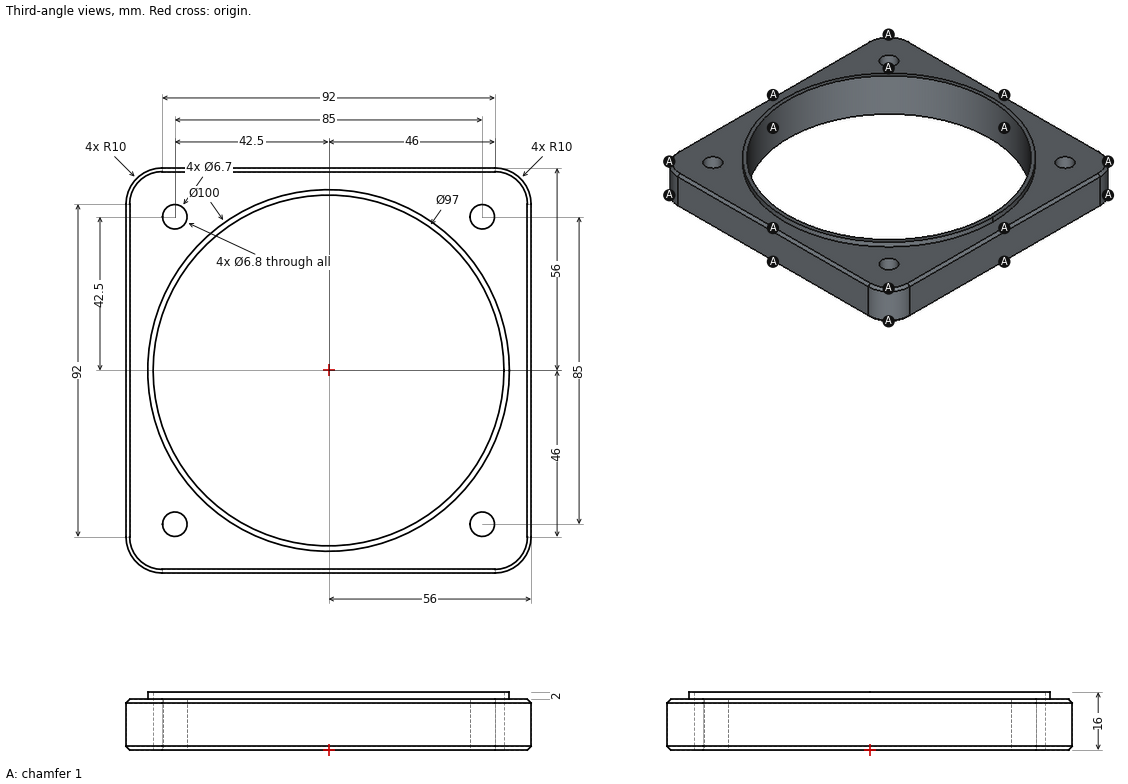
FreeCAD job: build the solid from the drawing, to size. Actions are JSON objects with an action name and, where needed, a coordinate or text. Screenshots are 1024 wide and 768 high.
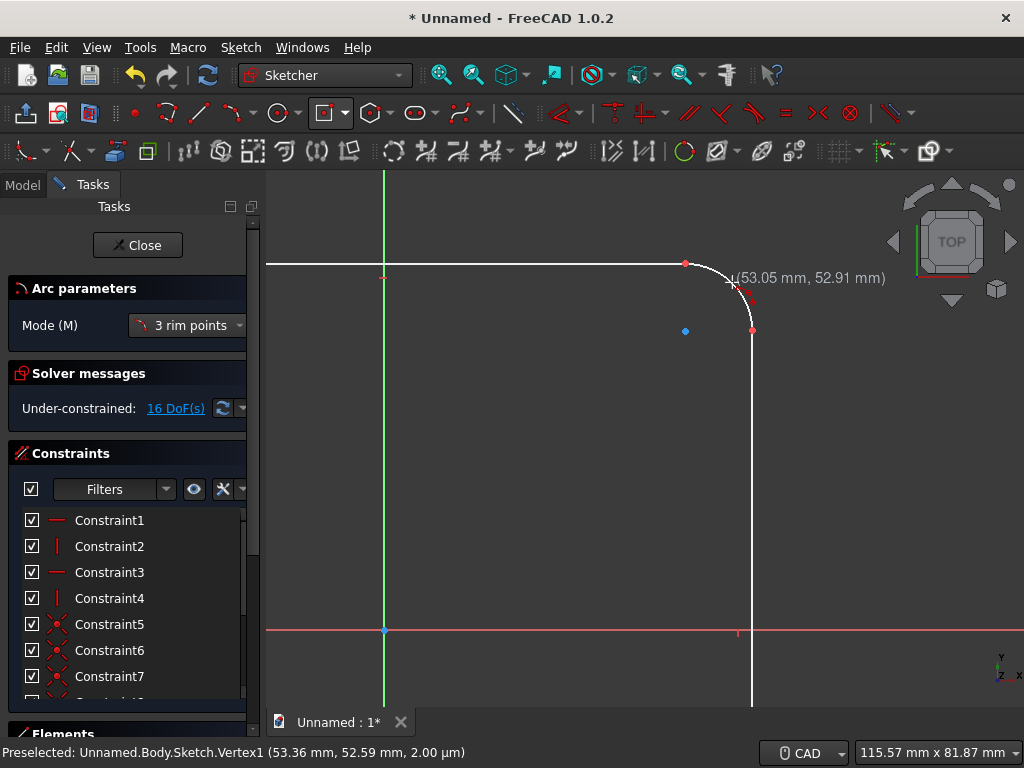
{"action": "left_click", "coordinate": [278, 114]}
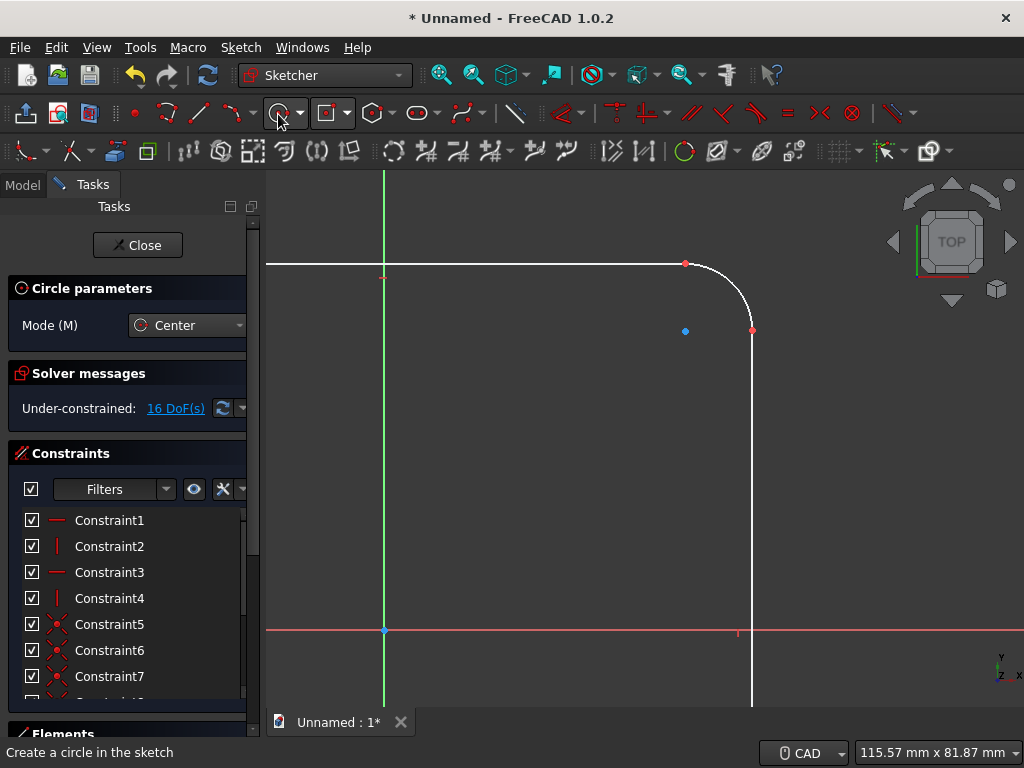
{"action": "left_click", "coordinate": [384, 630]}
{"action": "mouse_move", "coordinate": [609, 405]}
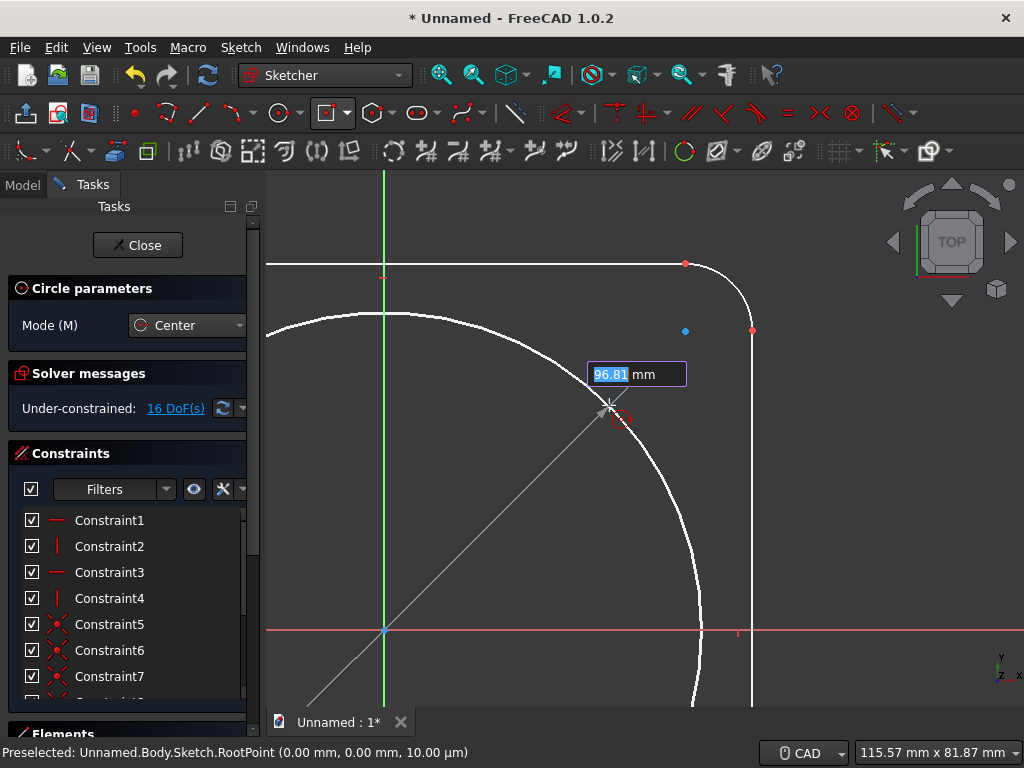
{"action": "type", "text": "97"}
{"action": "key", "text": "Return"}
{"action": "key", "text": "Escape"}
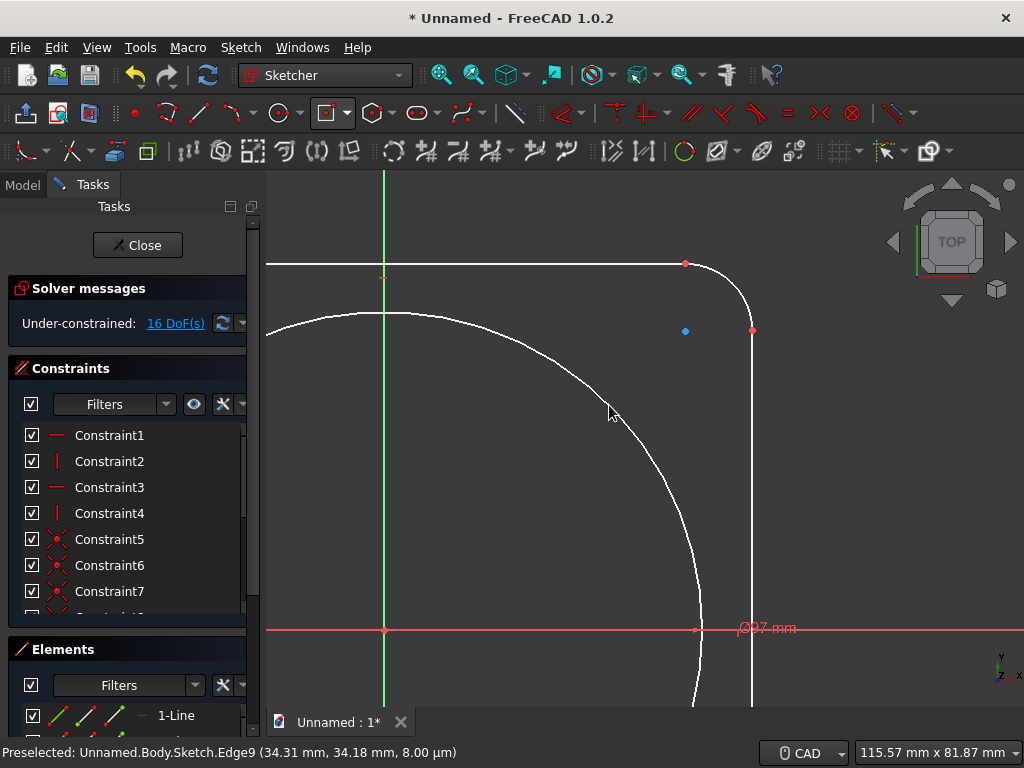
{"action": "left_click", "coordinate": [505, 264]}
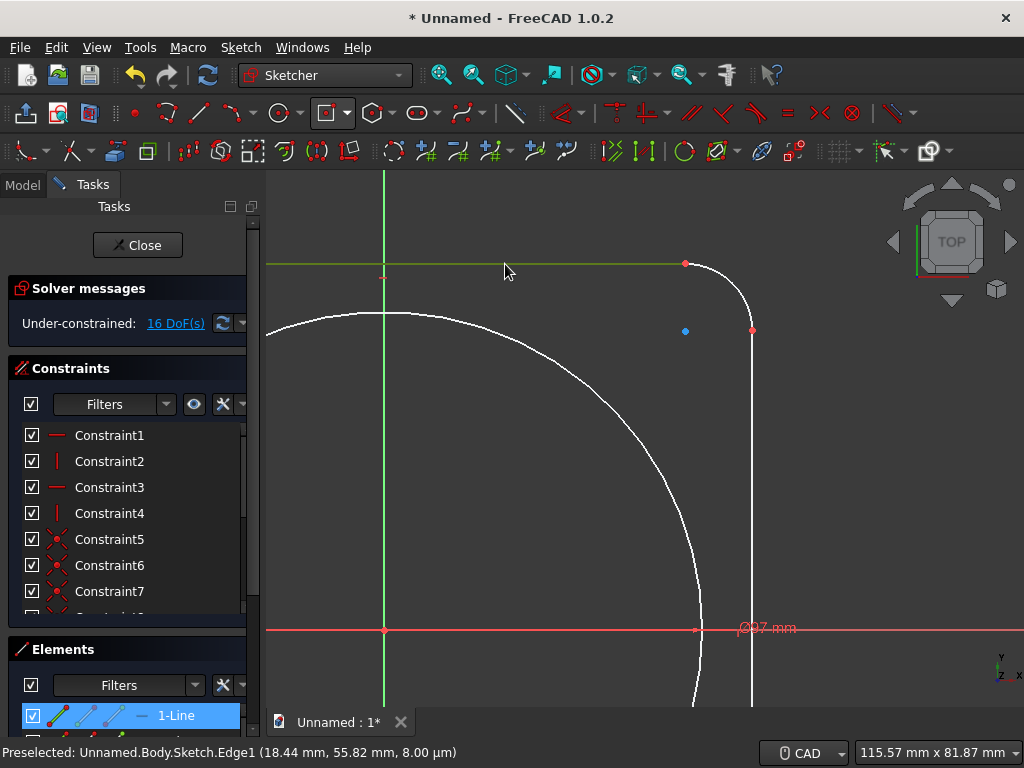
{"action": "scroll", "coordinate": [734, 282], "scroll_direction": "down", "scroll_amount": 4}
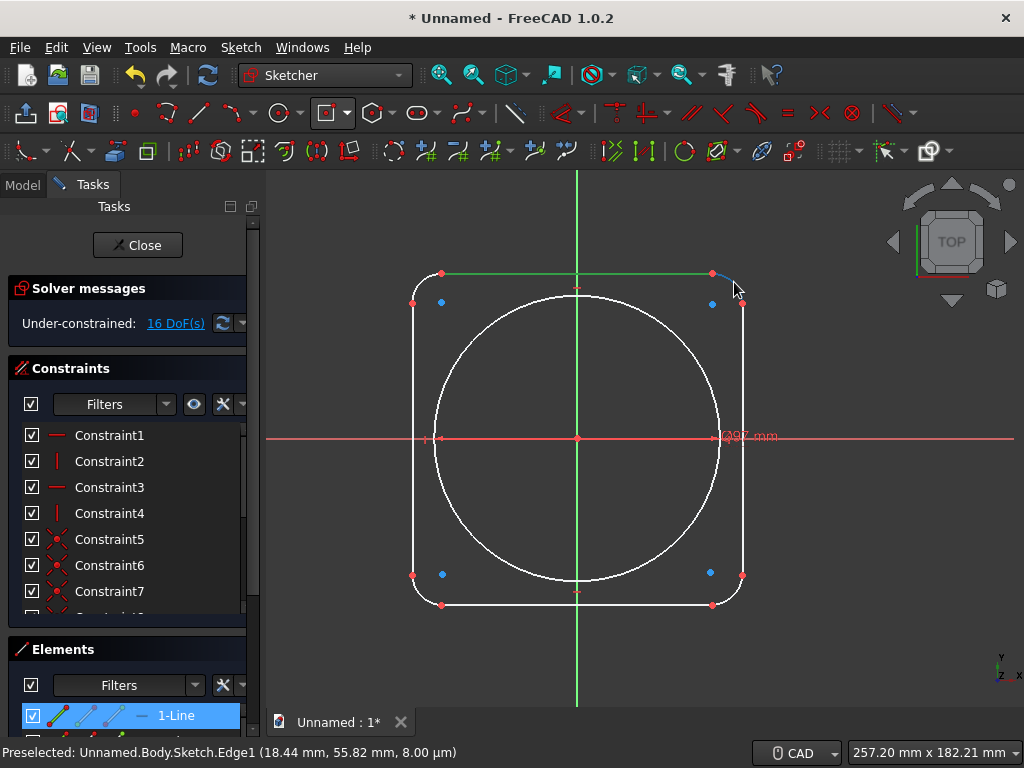
{"action": "left_click", "coordinate": [428, 277]}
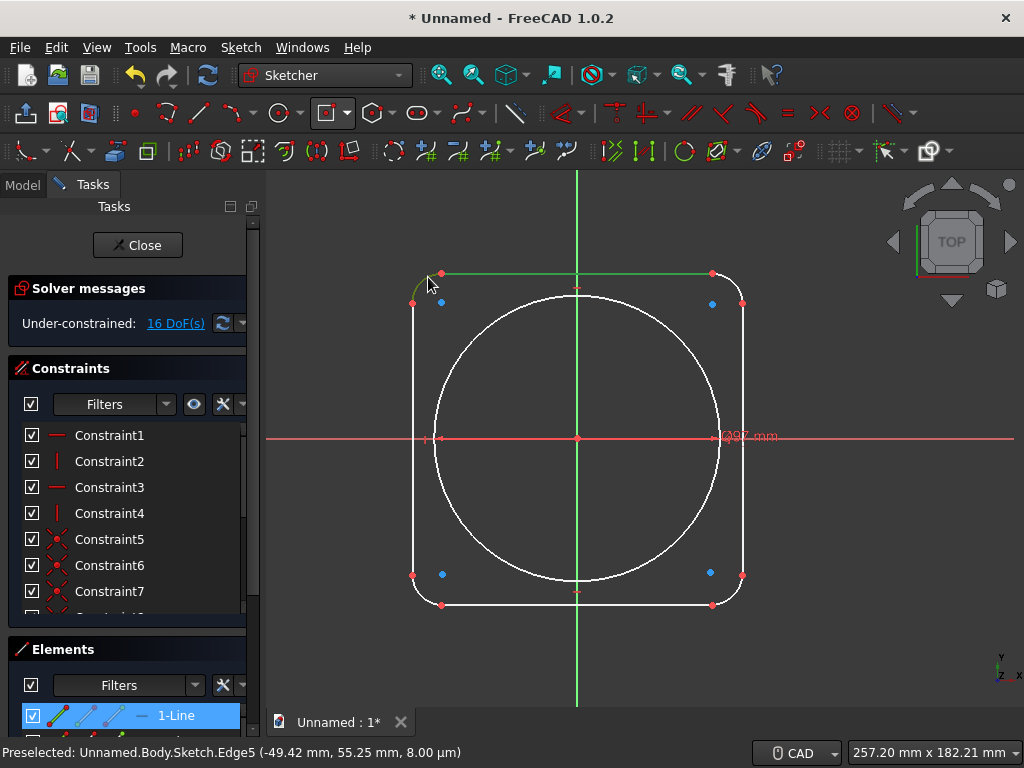
{"action": "left_click", "coordinate": [756, 114]}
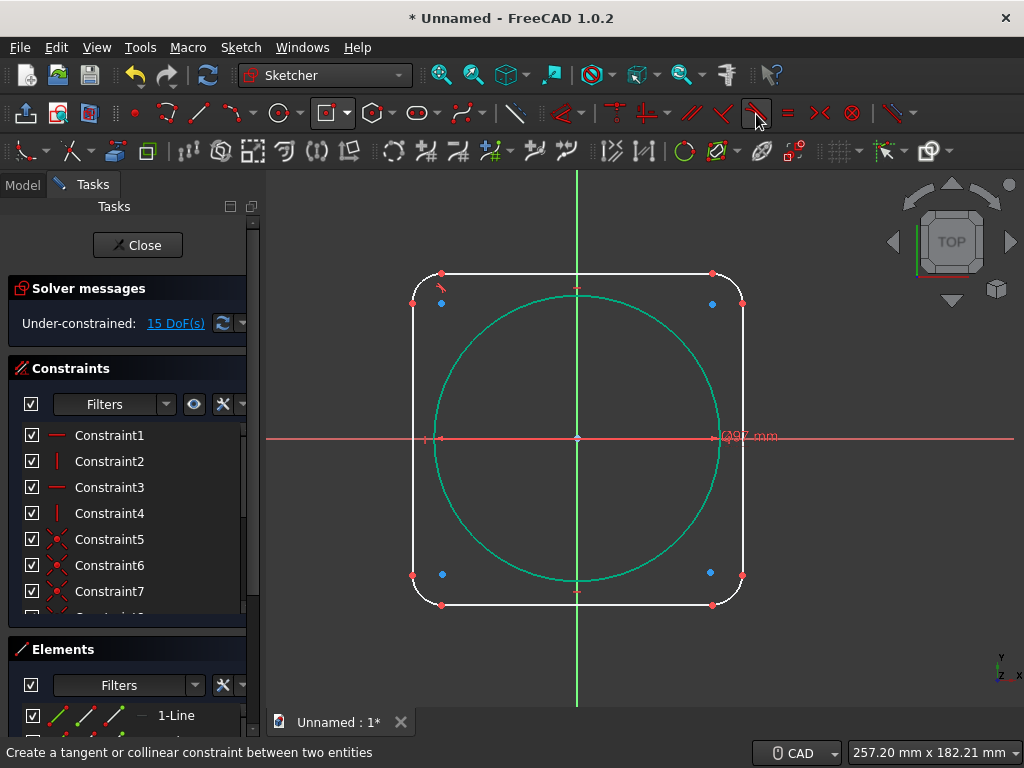
{"action": "left_click", "coordinate": [631, 274]}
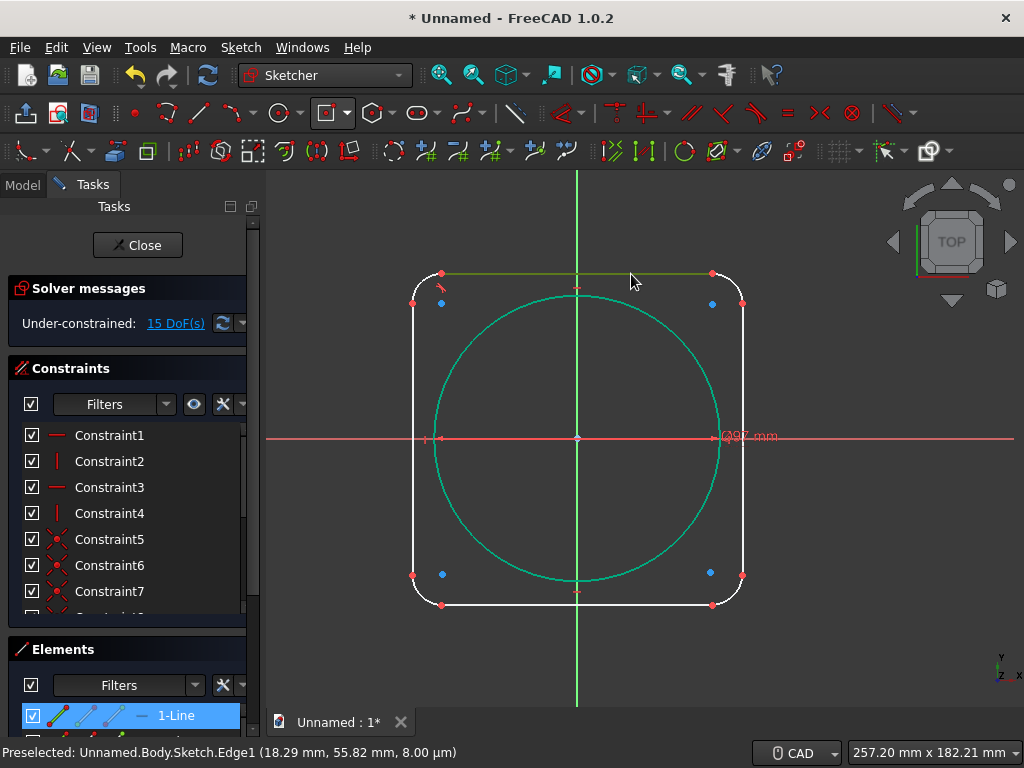
{"action": "left_click", "coordinate": [739, 290]}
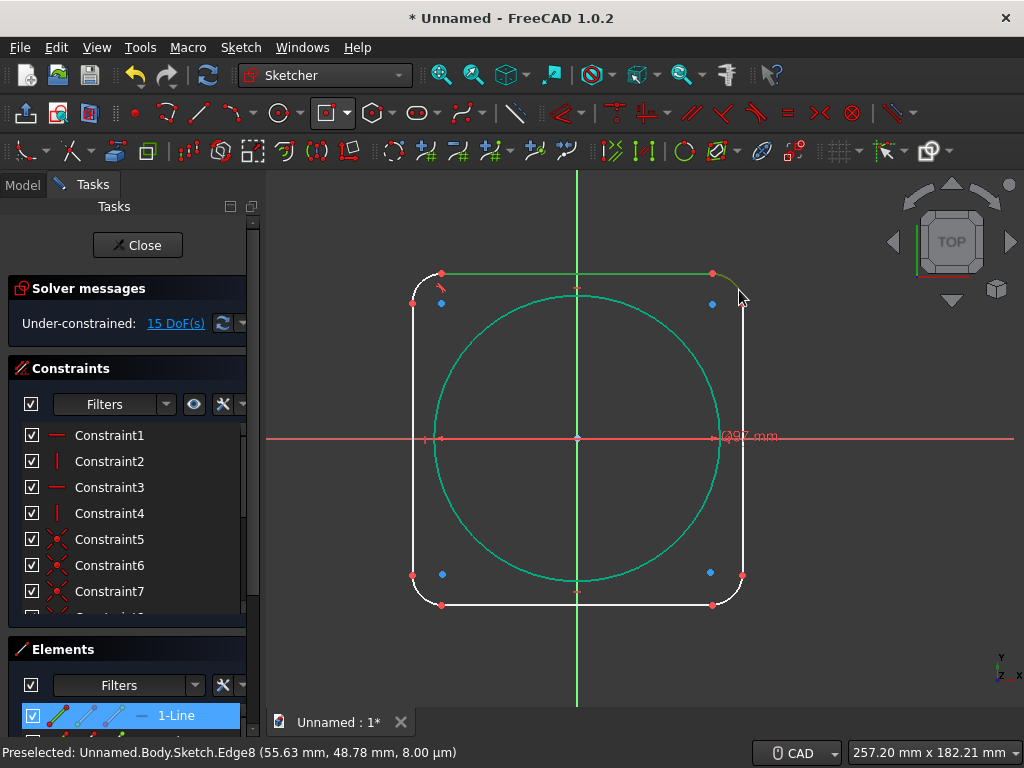
{"action": "left_click", "coordinate": [756, 114]}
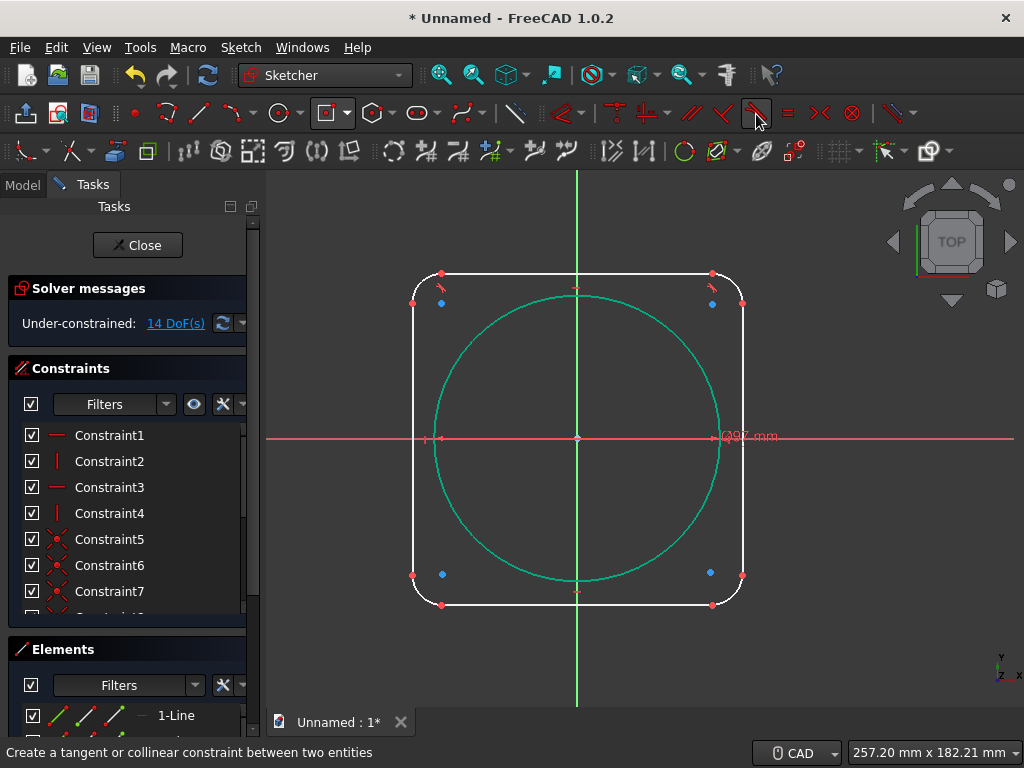
{"action": "left_click", "coordinate": [413, 385]}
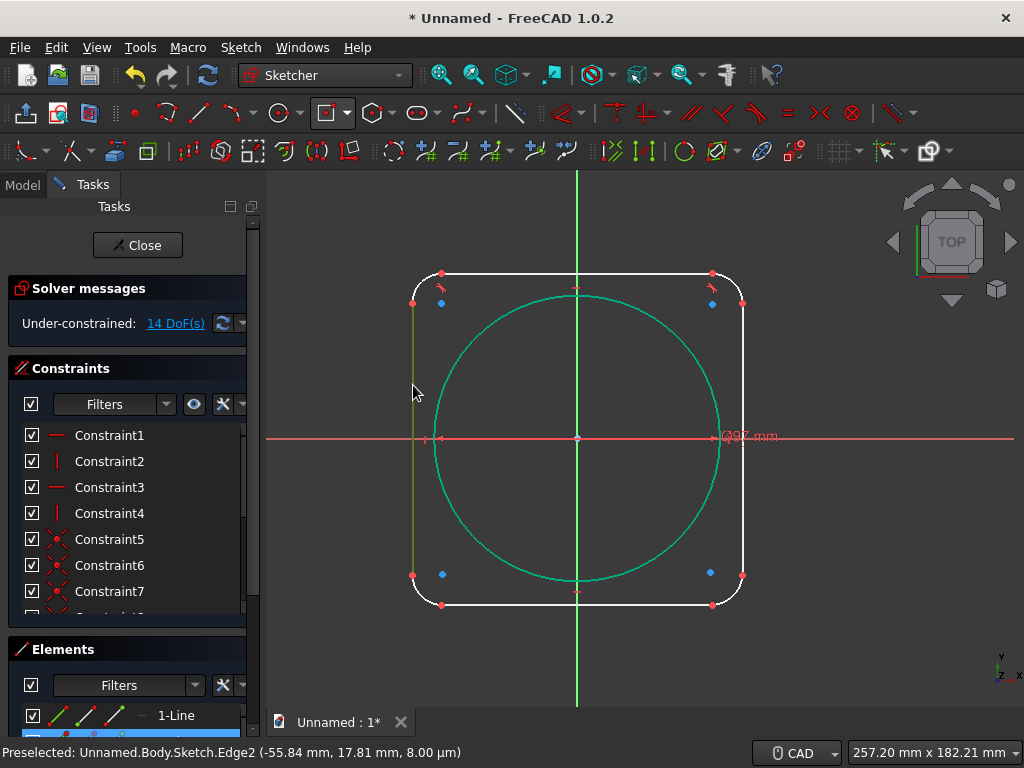
{"action": "left_click", "coordinate": [428, 277]}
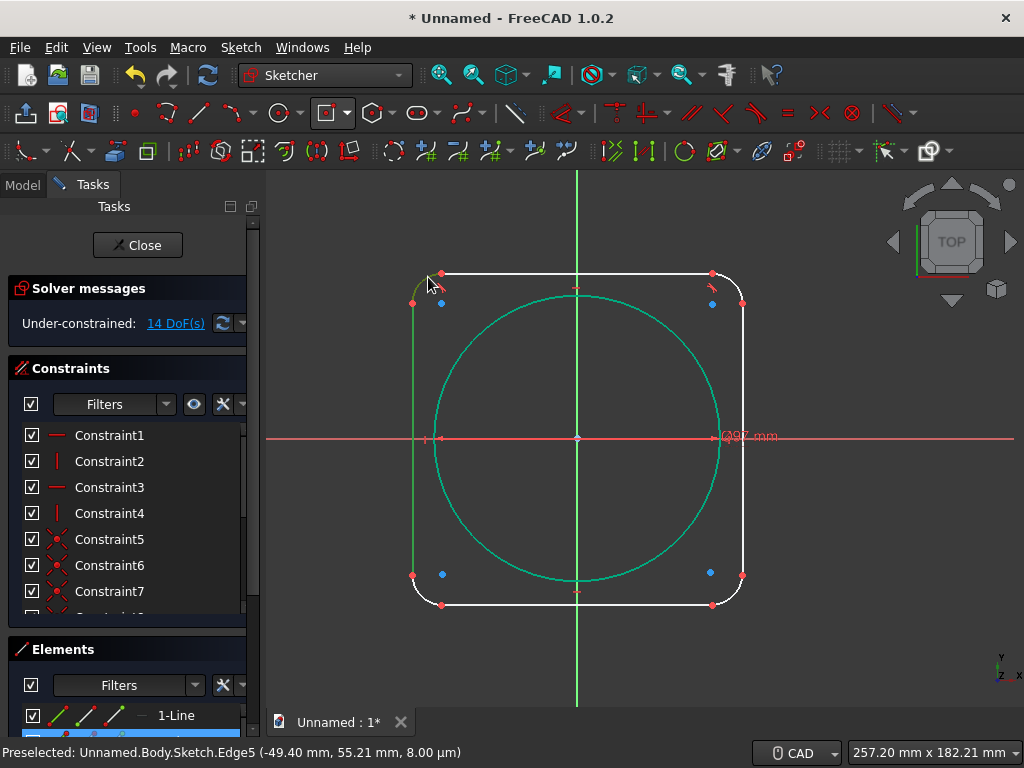
{"action": "left_click", "coordinate": [756, 114]}